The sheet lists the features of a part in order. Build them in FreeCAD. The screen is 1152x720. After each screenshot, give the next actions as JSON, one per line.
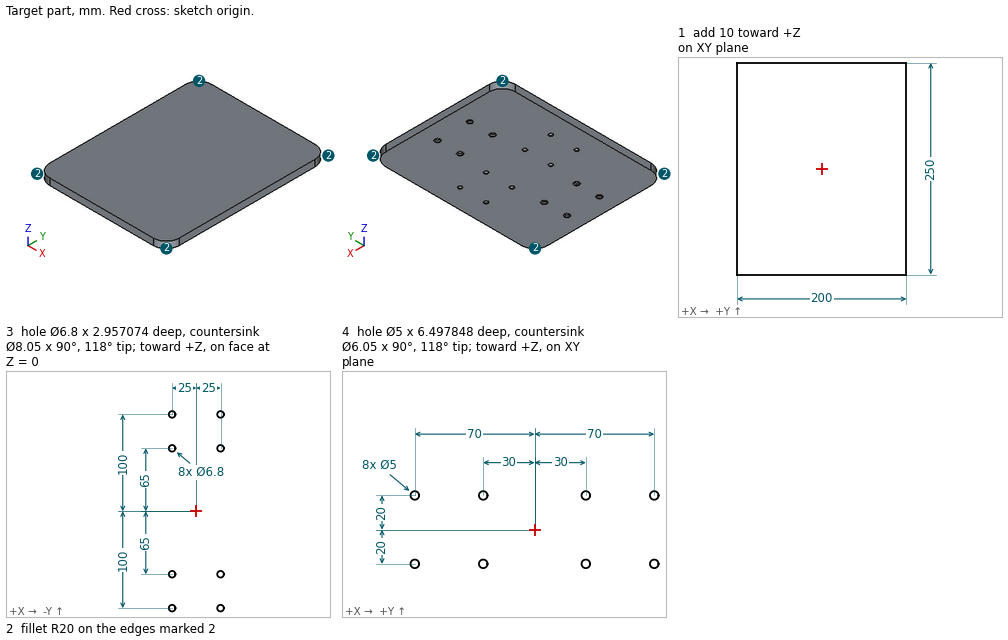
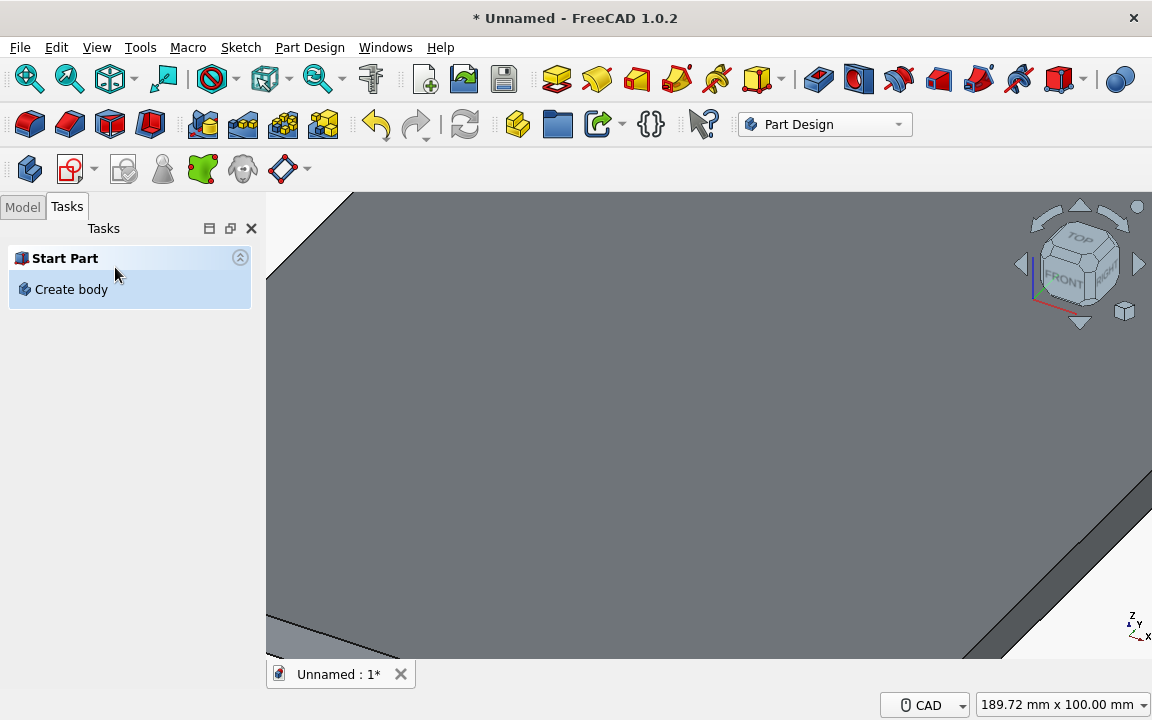
{"action": "key", "text": "v f"}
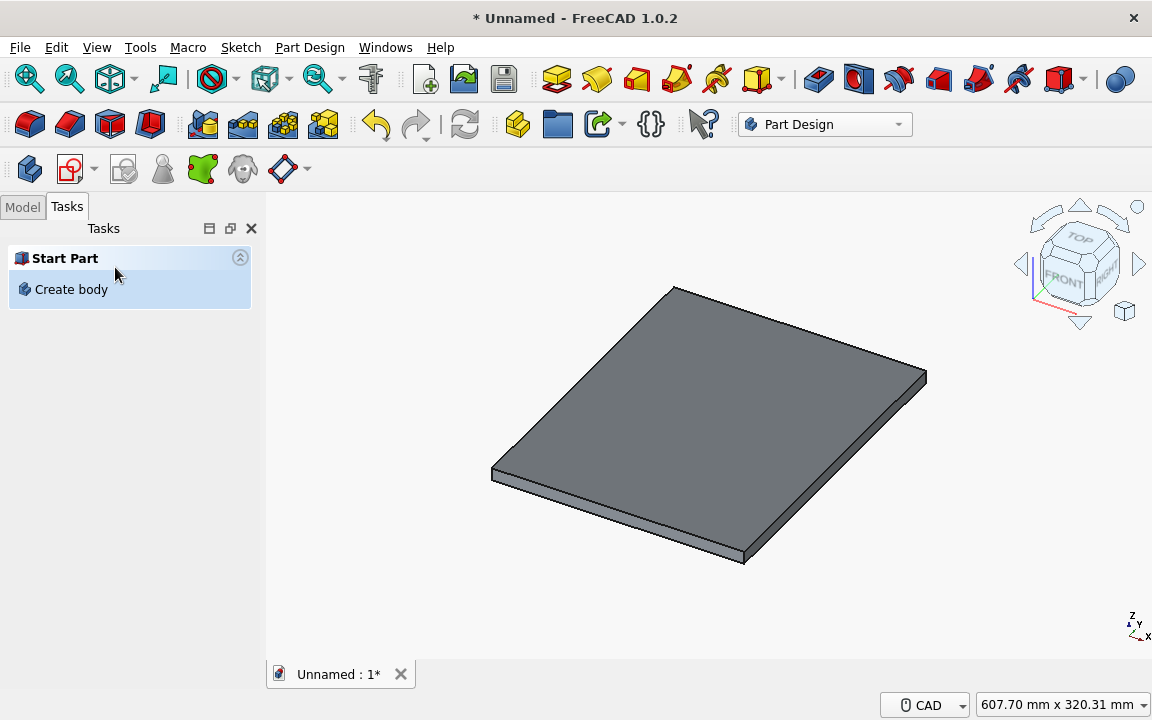
{"action": "left_click", "coordinate": [744, 557]}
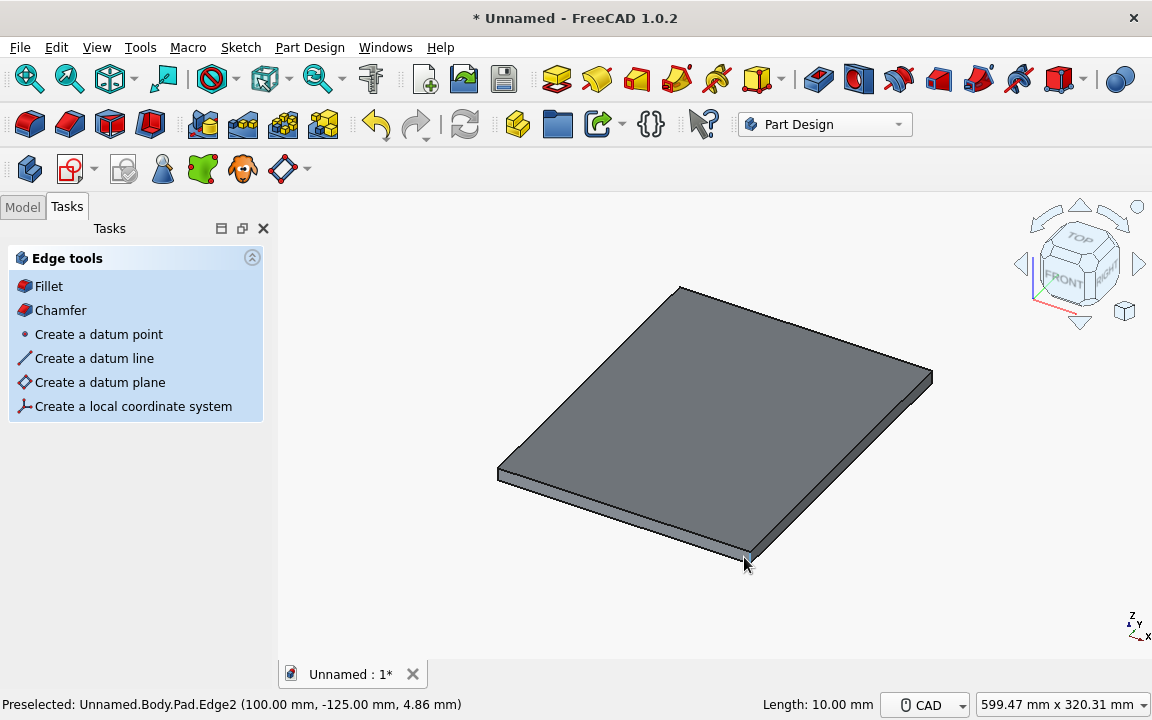
{"action": "scroll", "coordinate": [680, 292], "scroll_direction": "up", "scroll_amount": 6}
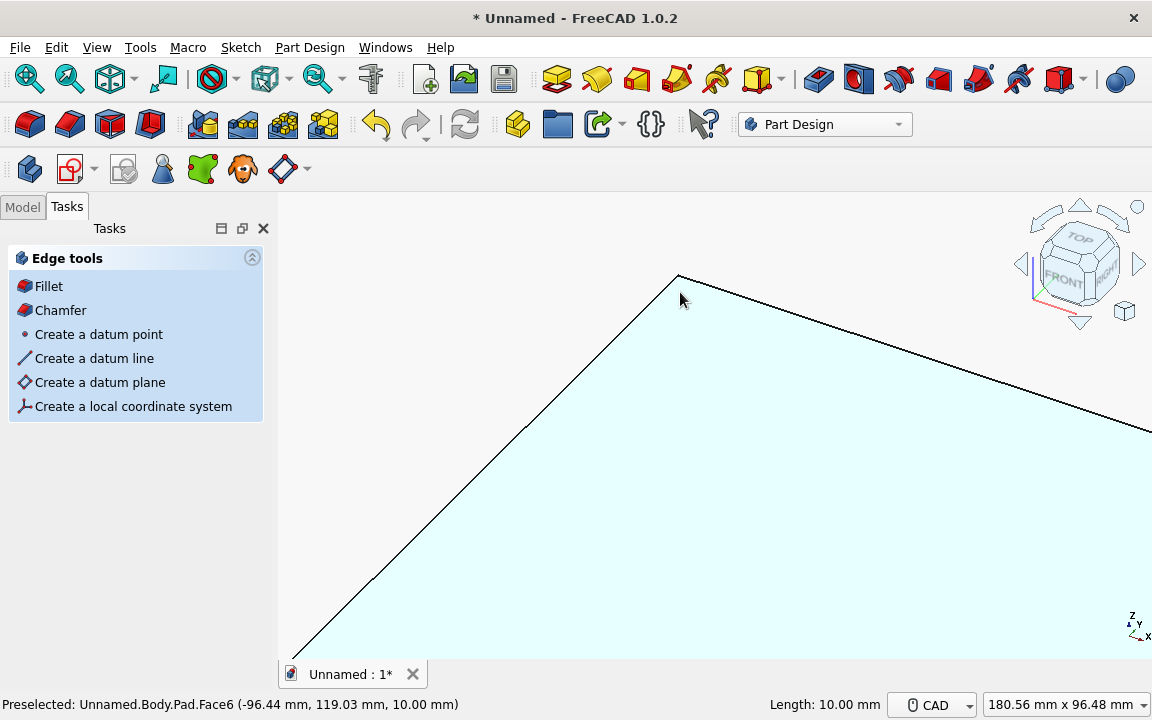
{"action": "key", "text": "v f"}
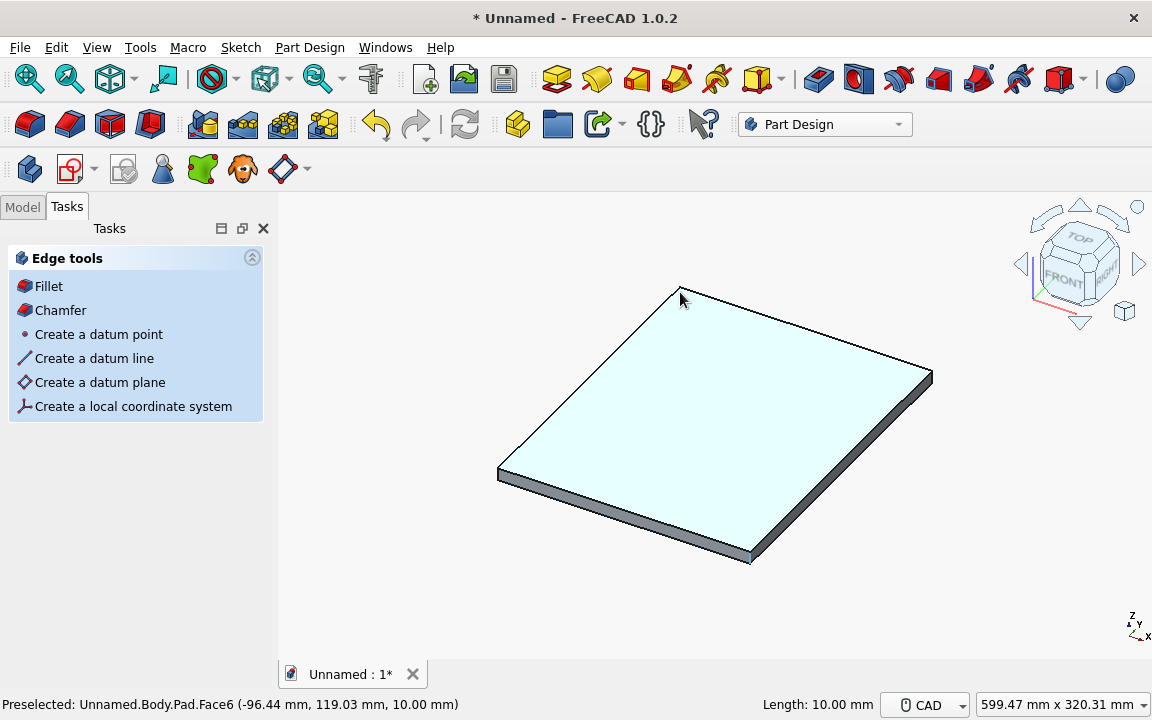
{"action": "key", "text": "0"}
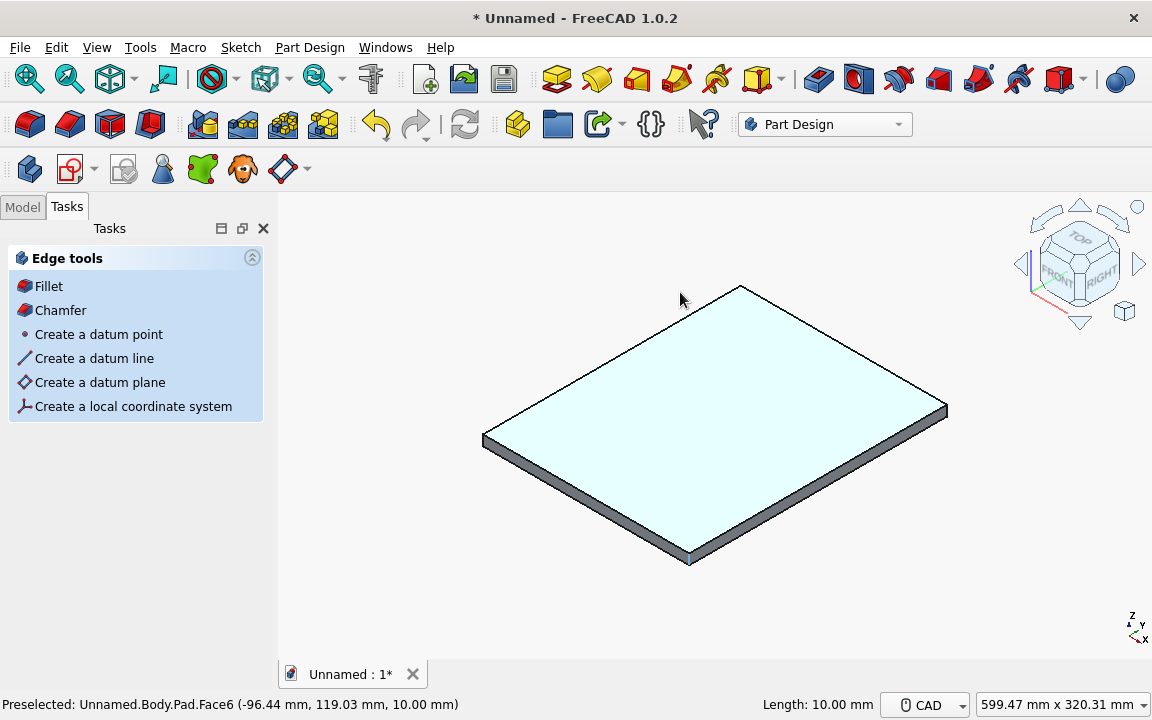
{"action": "scroll", "coordinate": [741, 291], "scroll_direction": "up", "scroll_amount": 6}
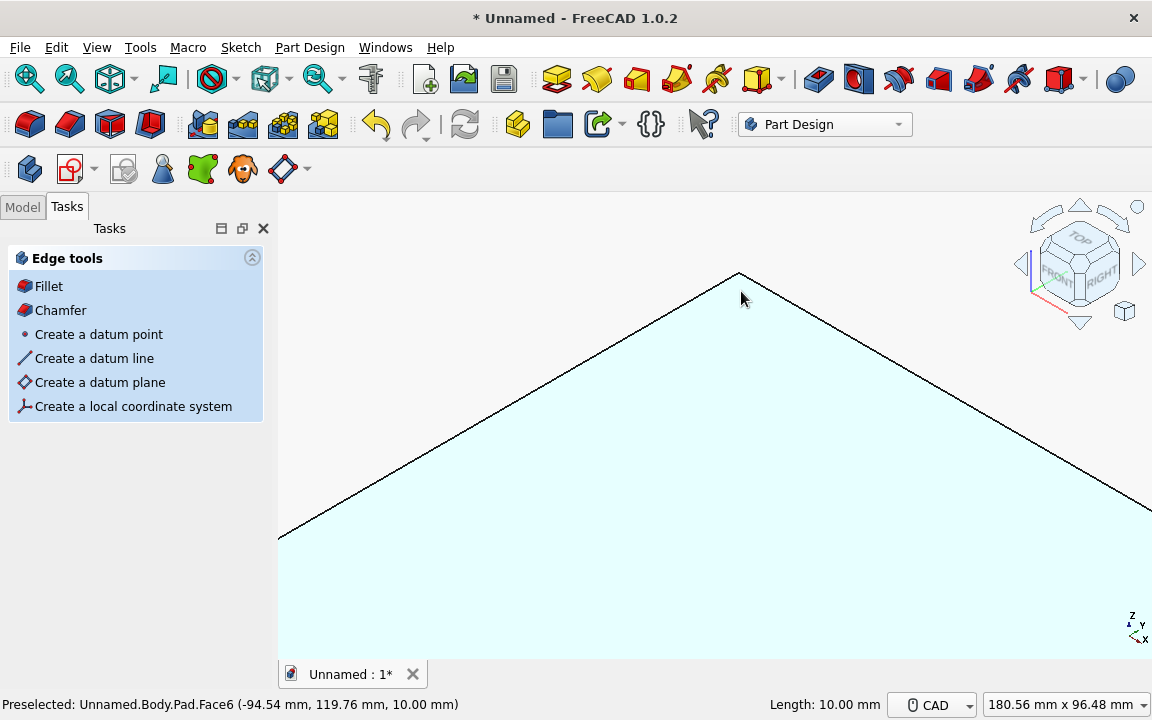
{"action": "key", "text": "v f"}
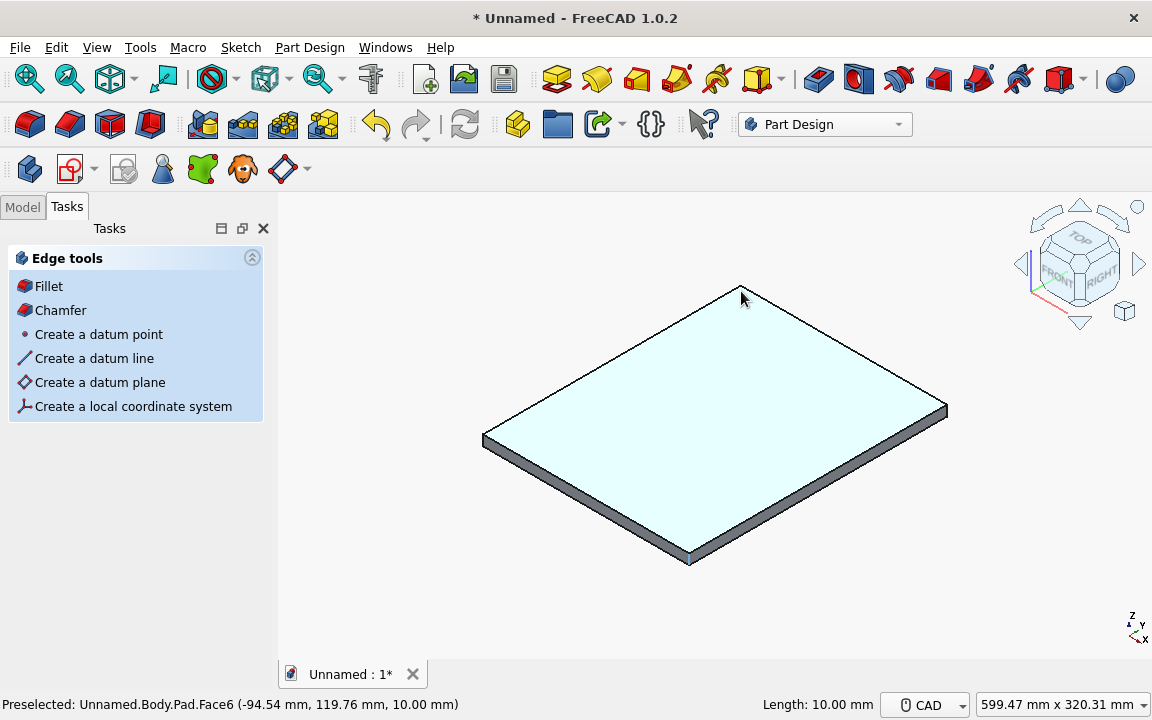
{"action": "key", "text": "2"}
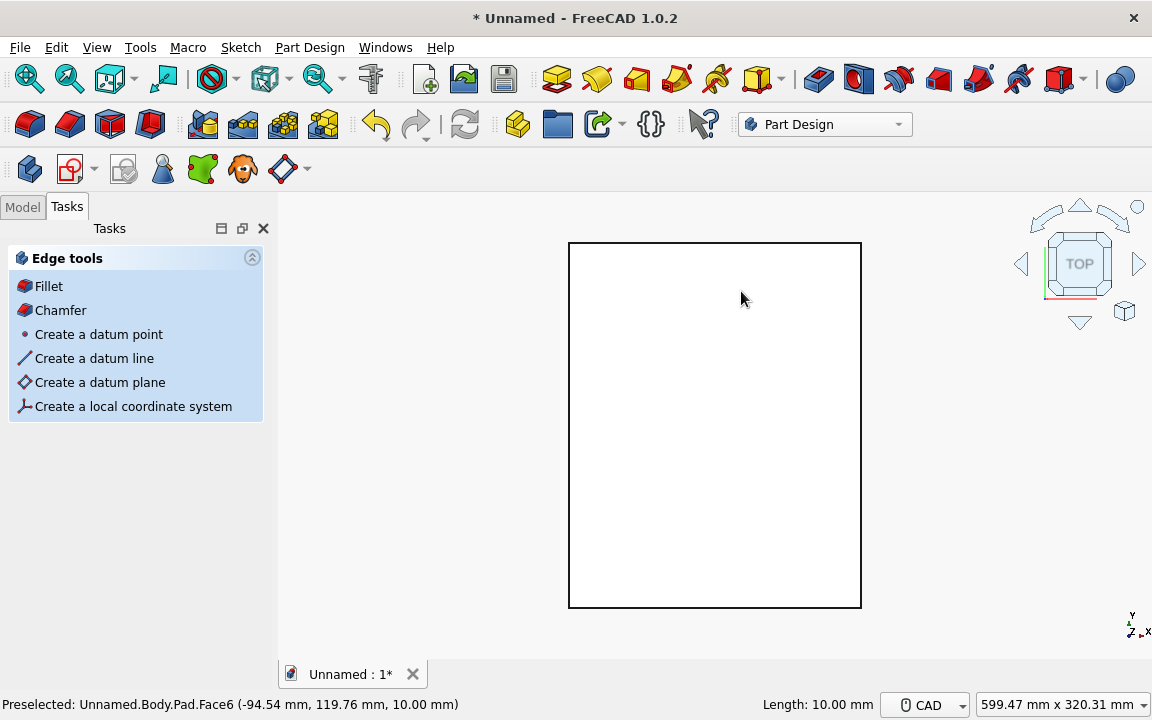
{"action": "scroll", "coordinate": [569, 242], "scroll_direction": "up", "scroll_amount": 6}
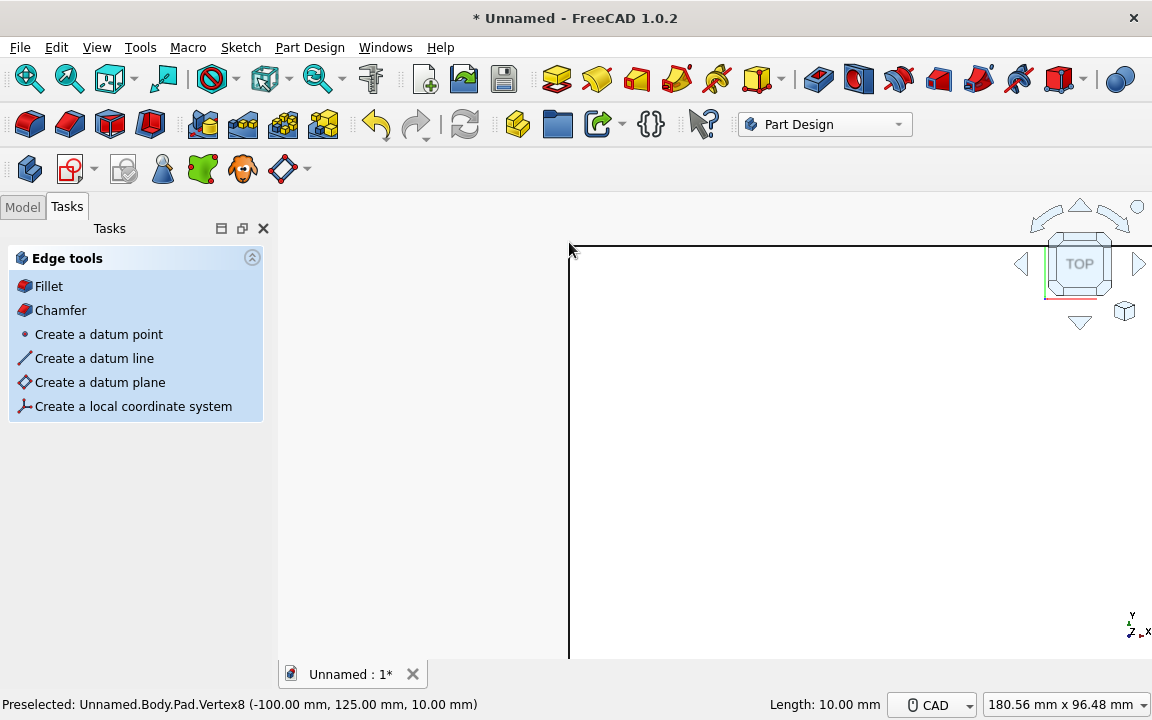
{"action": "left_click", "coordinate": [30, 80]}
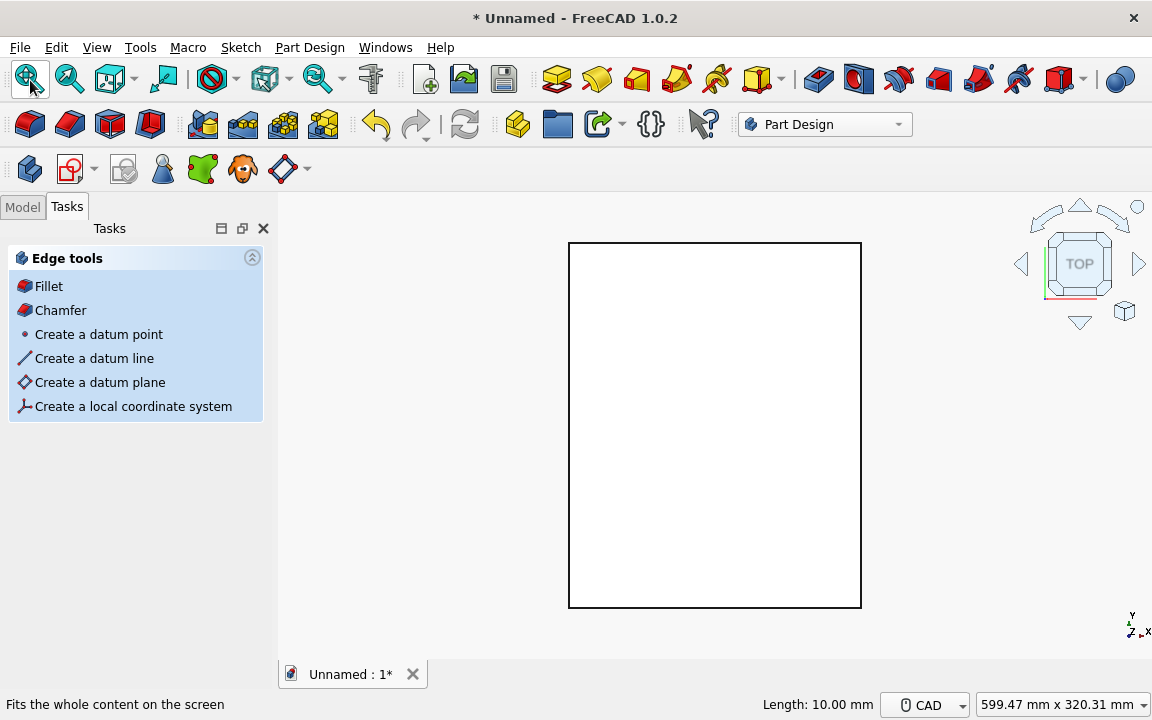
{"action": "key", "text": "1"}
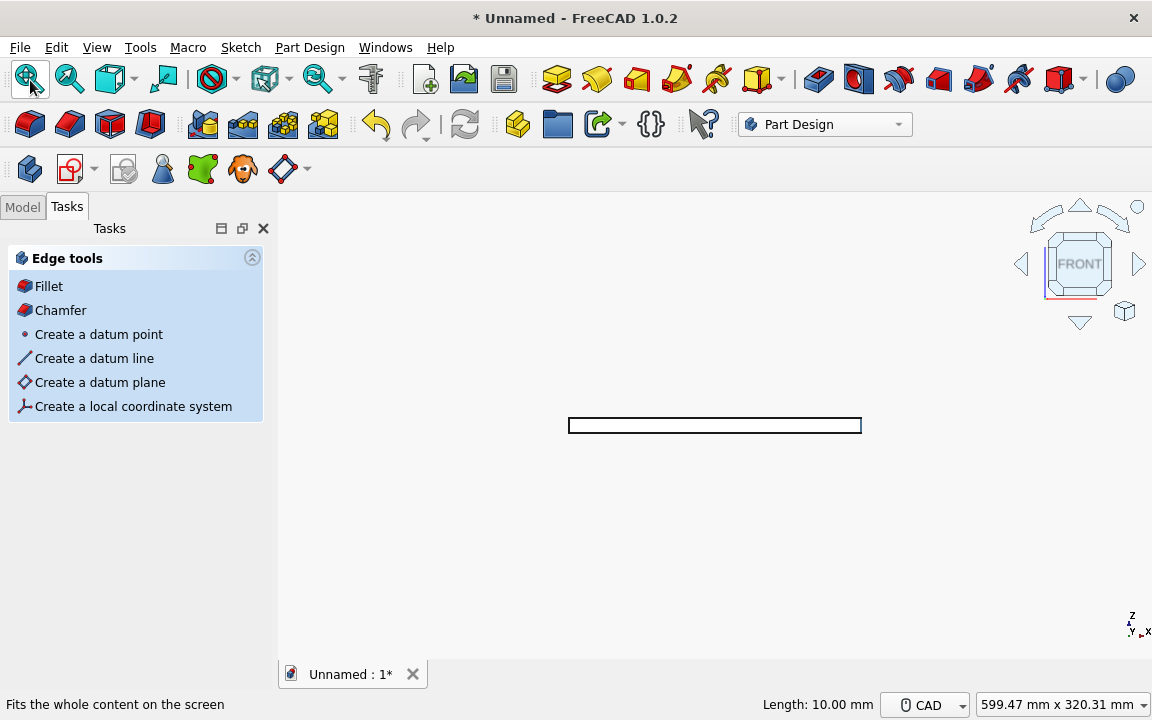
{"action": "key", "text": "v f"}